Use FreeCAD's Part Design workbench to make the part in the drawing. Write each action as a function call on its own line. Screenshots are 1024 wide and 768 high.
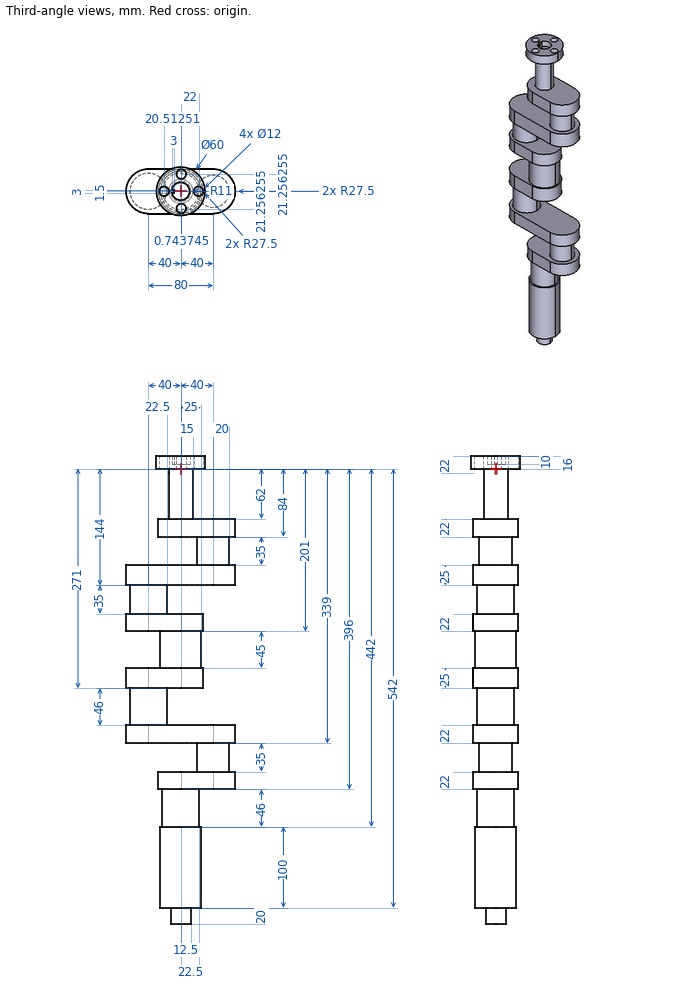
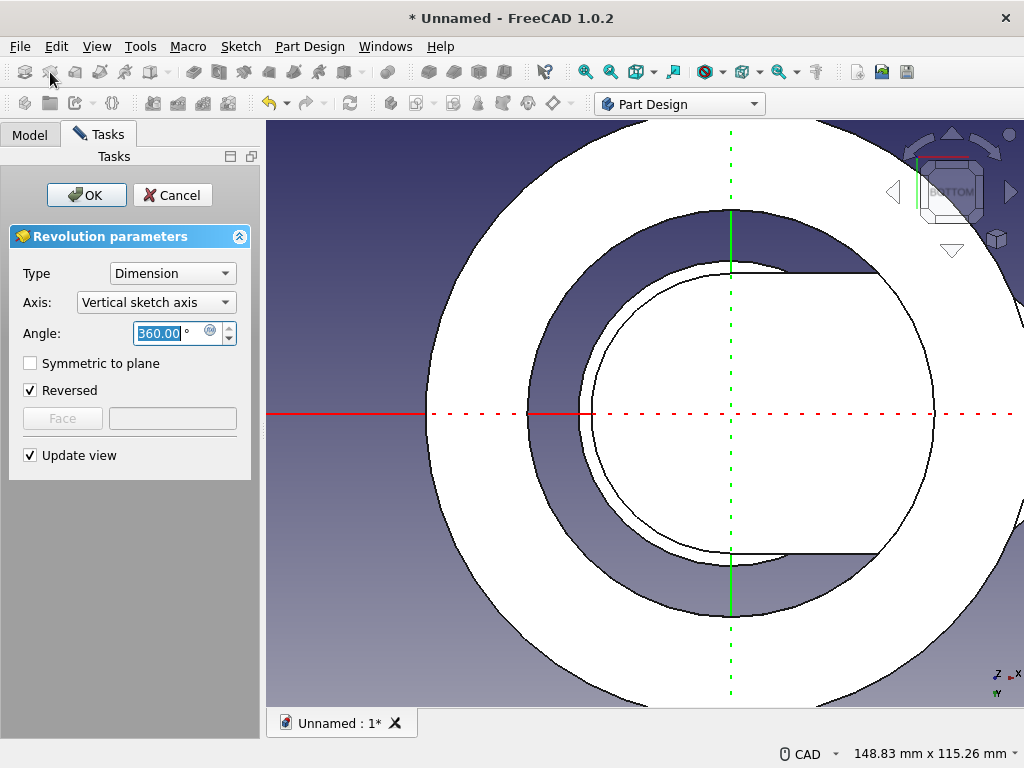
click(157, 302)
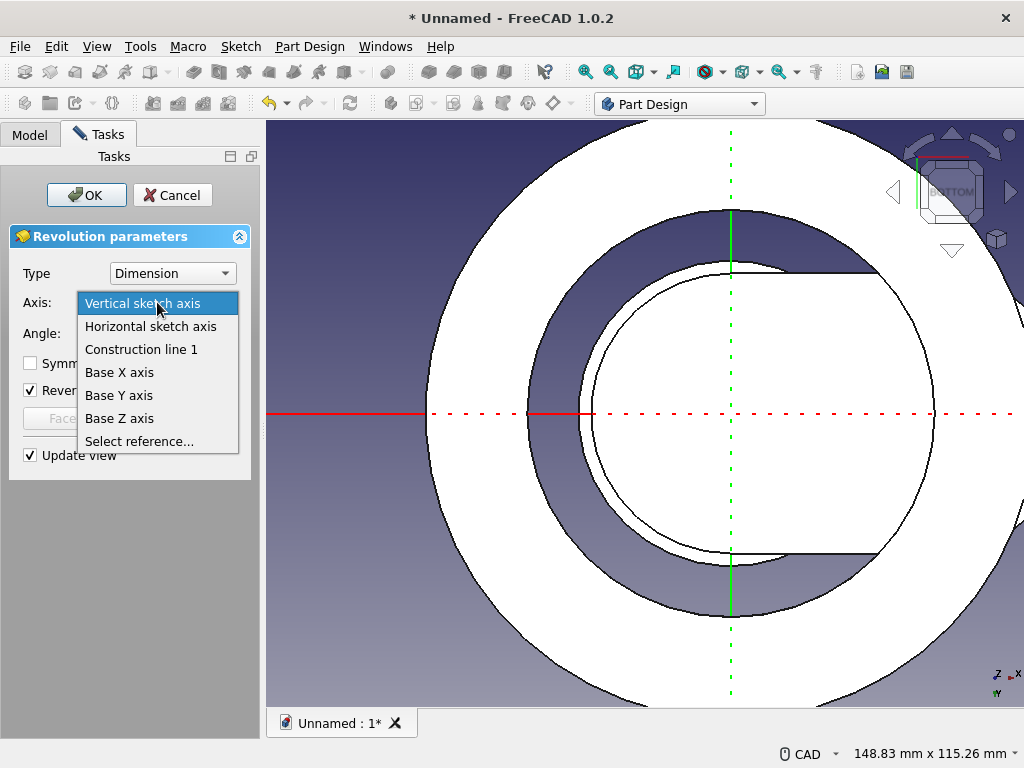
click(156, 350)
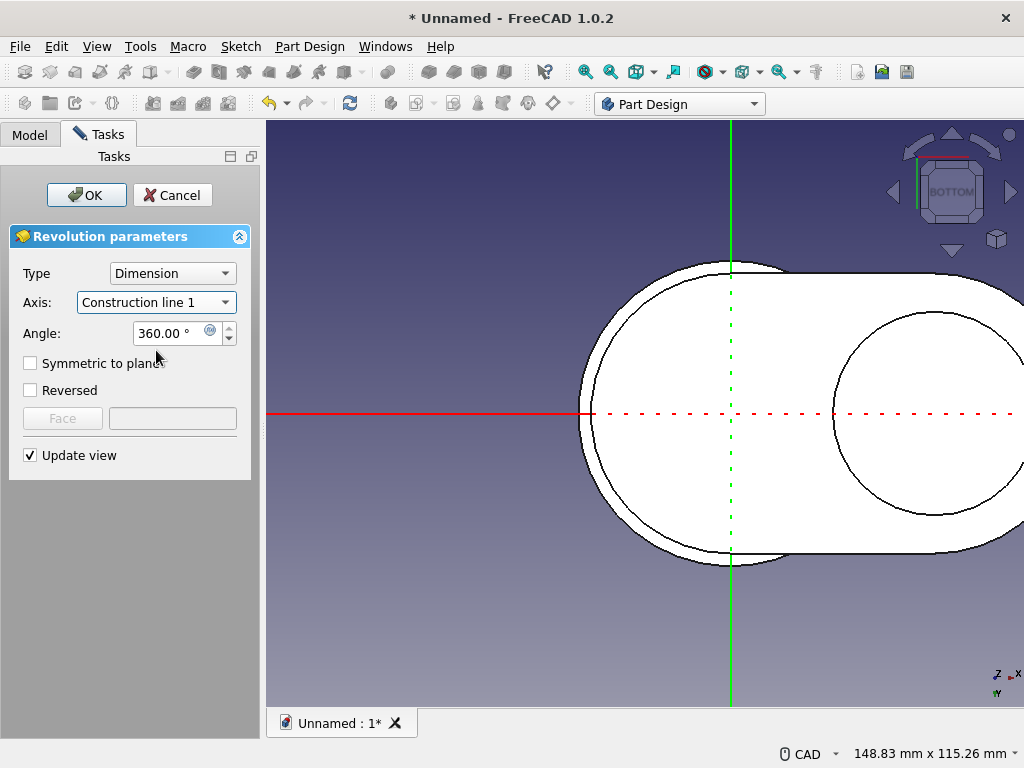
click(87, 195)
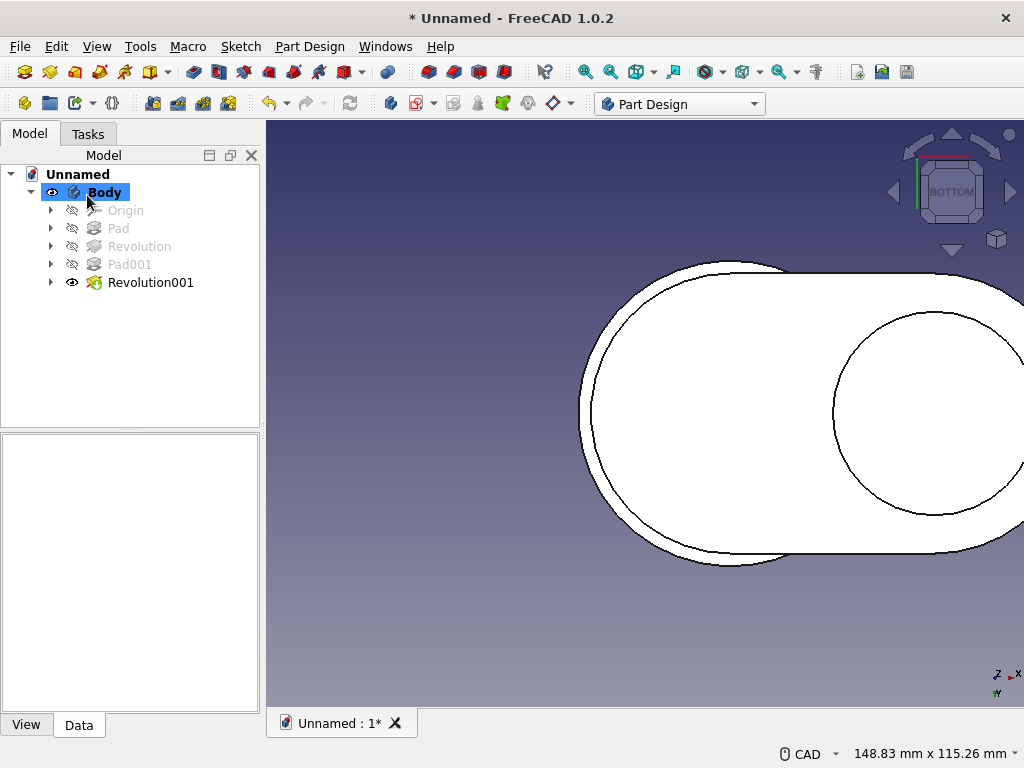
key(v)
key(f)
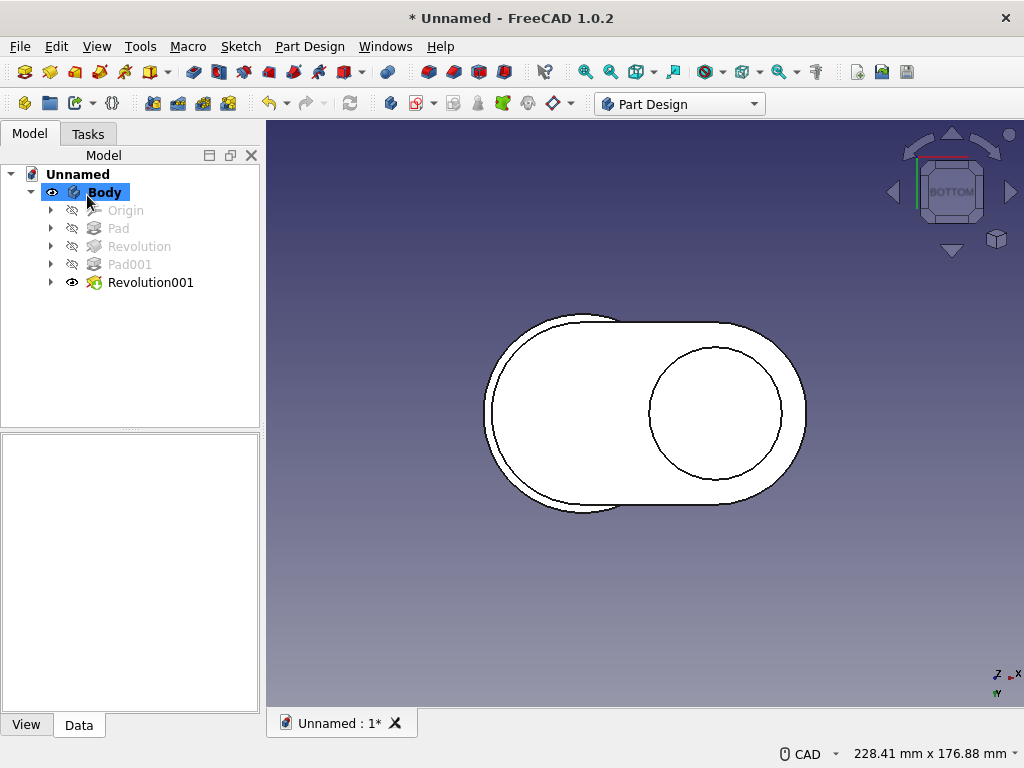
click(716, 412)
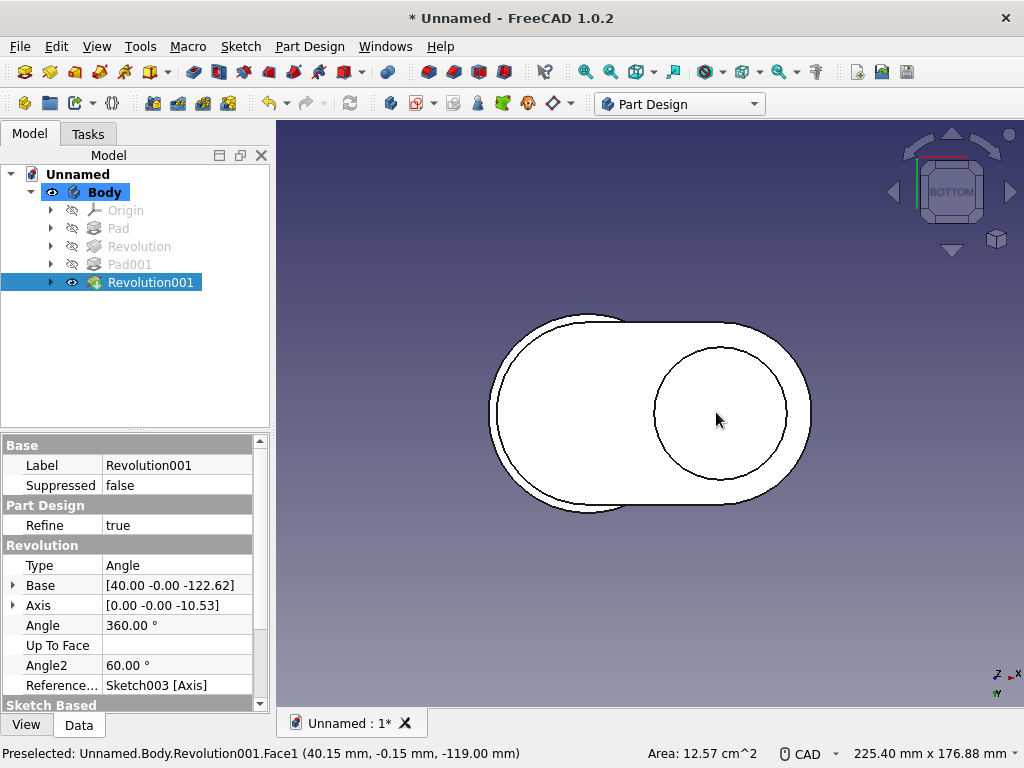
click(416, 104)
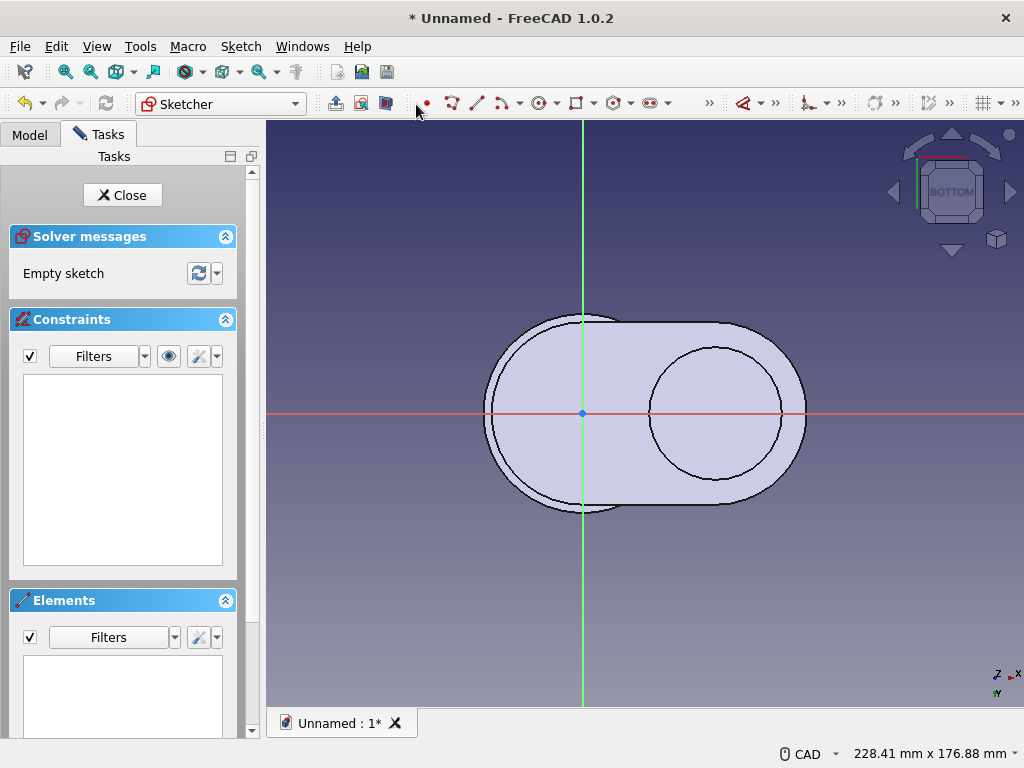
key(g)
key(s)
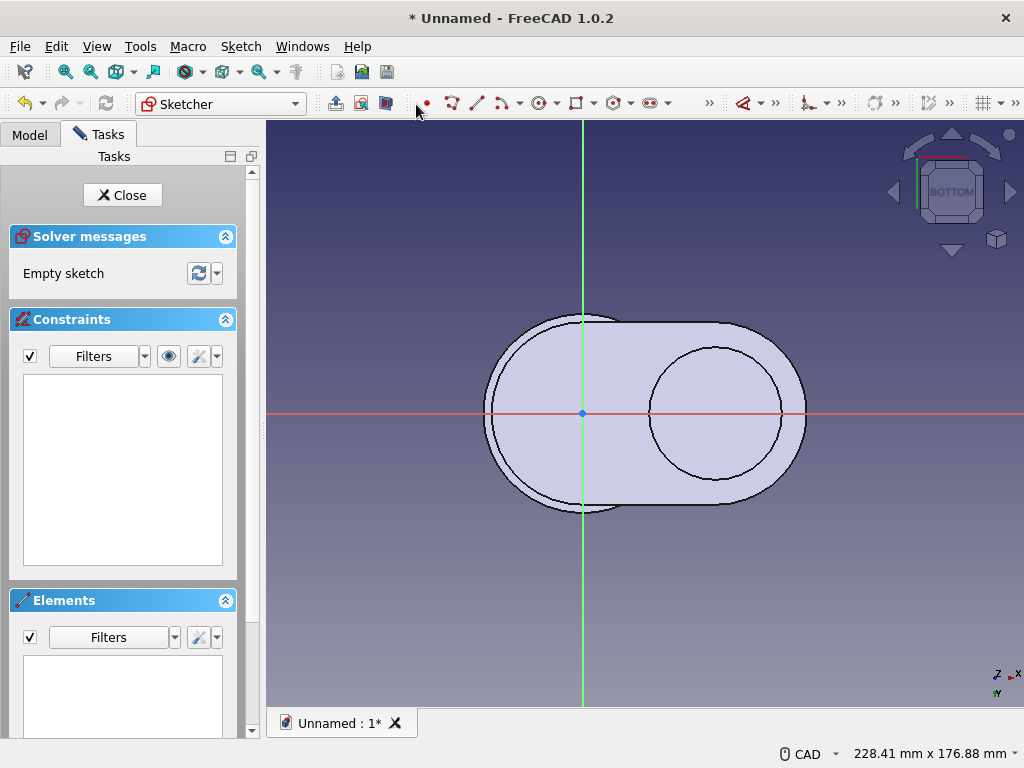
click(450, 413)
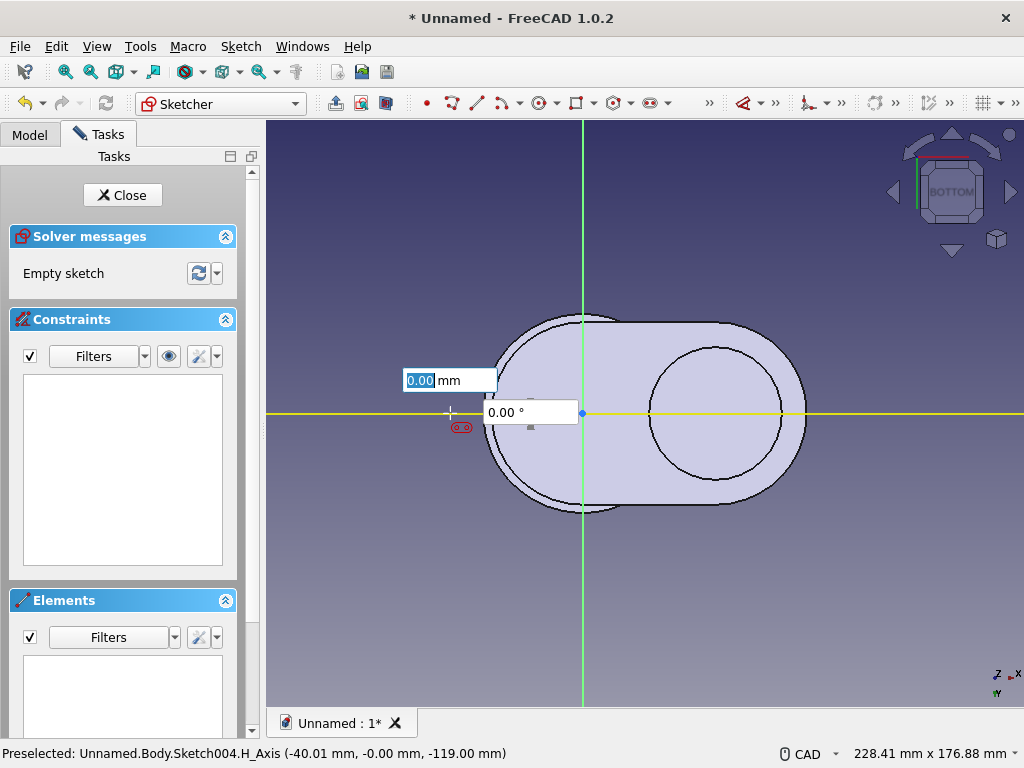
click(716, 404)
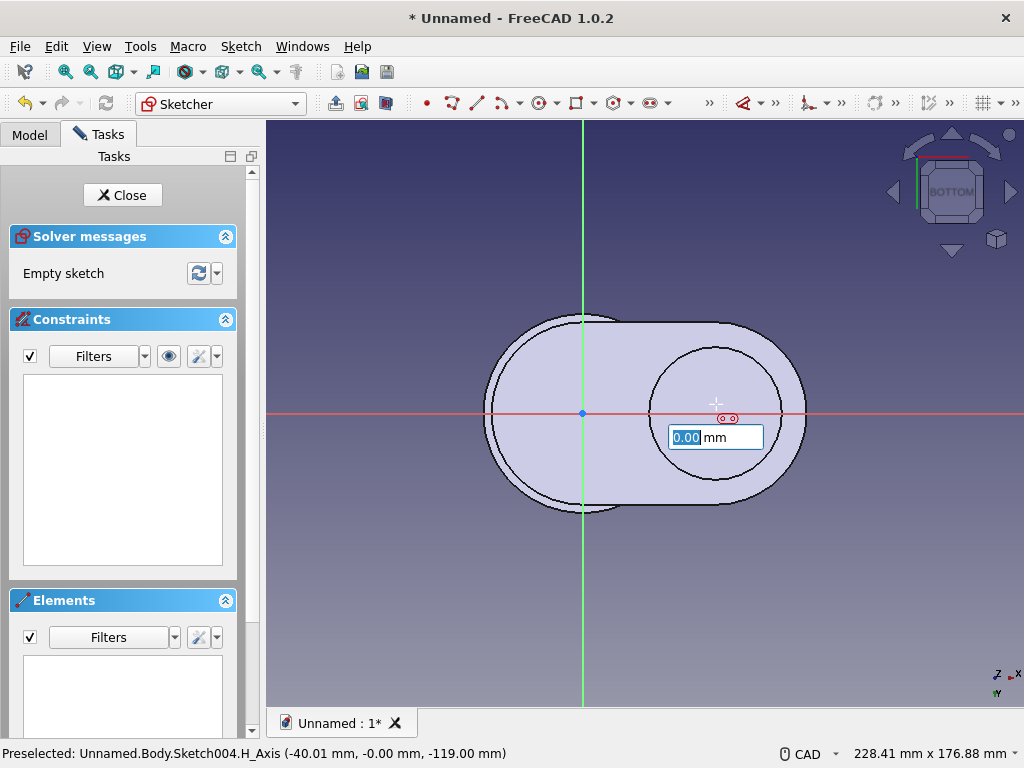
click(543, 505)
key(Escape)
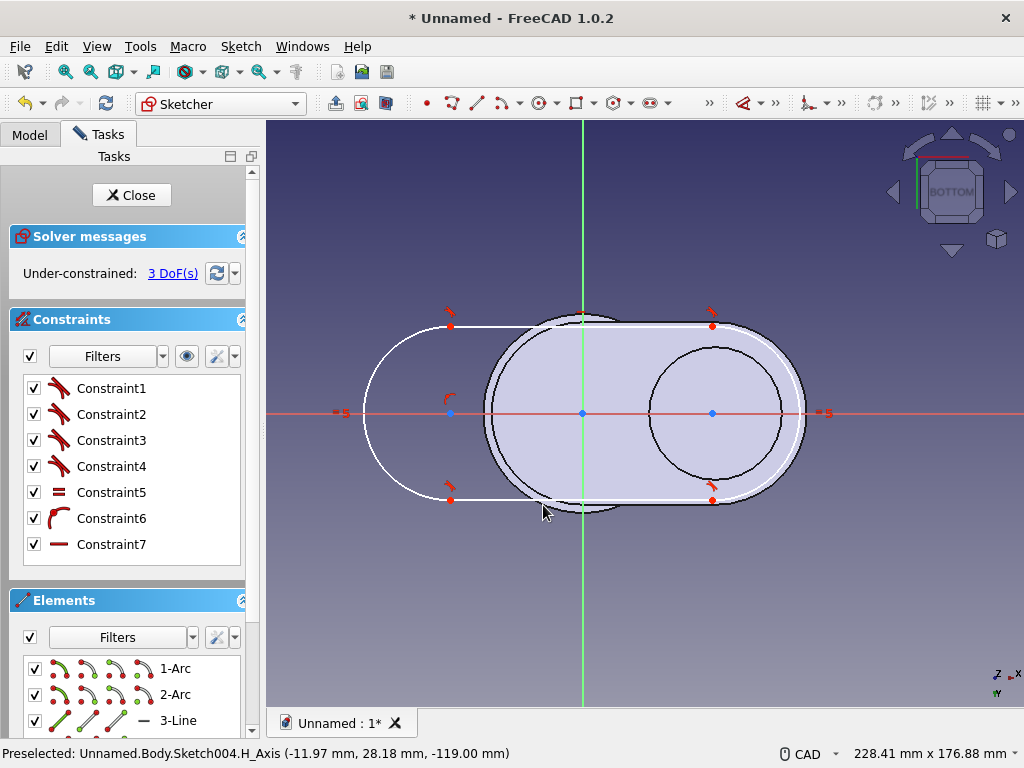
key(d)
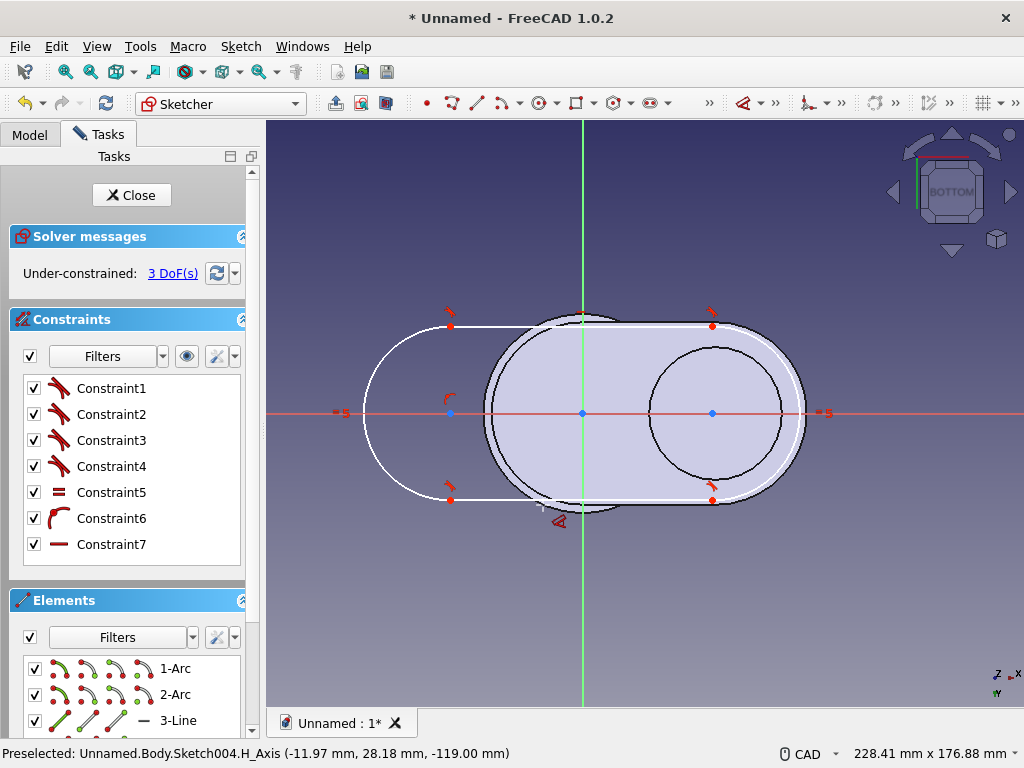
click(380, 362)
click(354, 343)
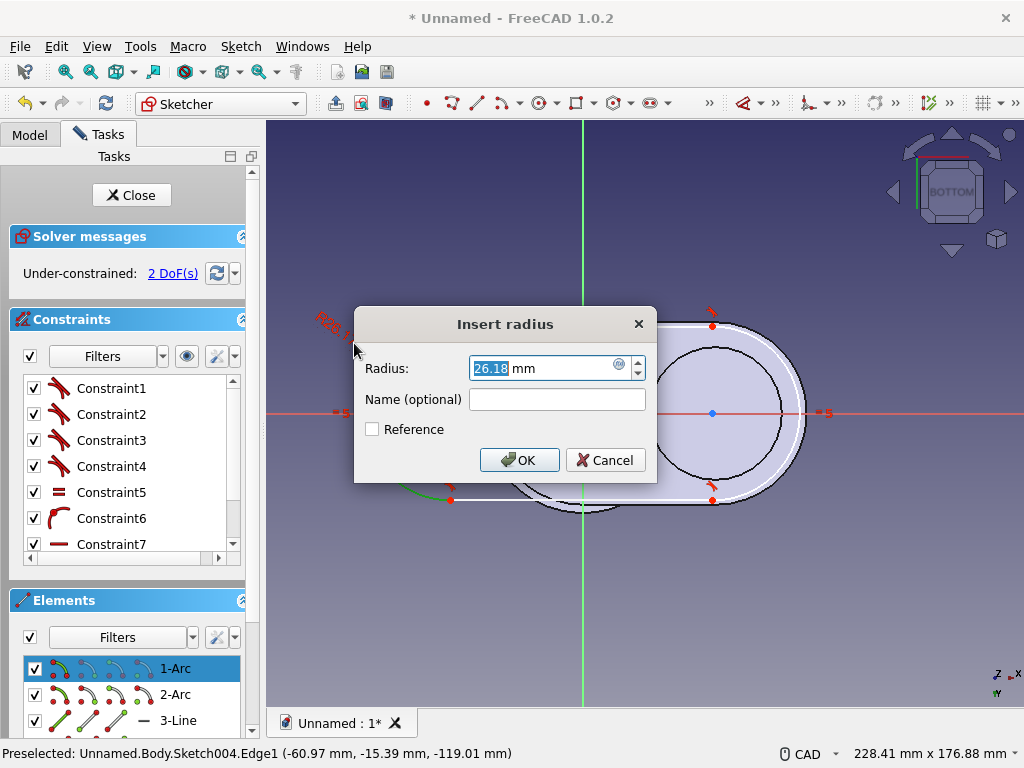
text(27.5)
key(Return)